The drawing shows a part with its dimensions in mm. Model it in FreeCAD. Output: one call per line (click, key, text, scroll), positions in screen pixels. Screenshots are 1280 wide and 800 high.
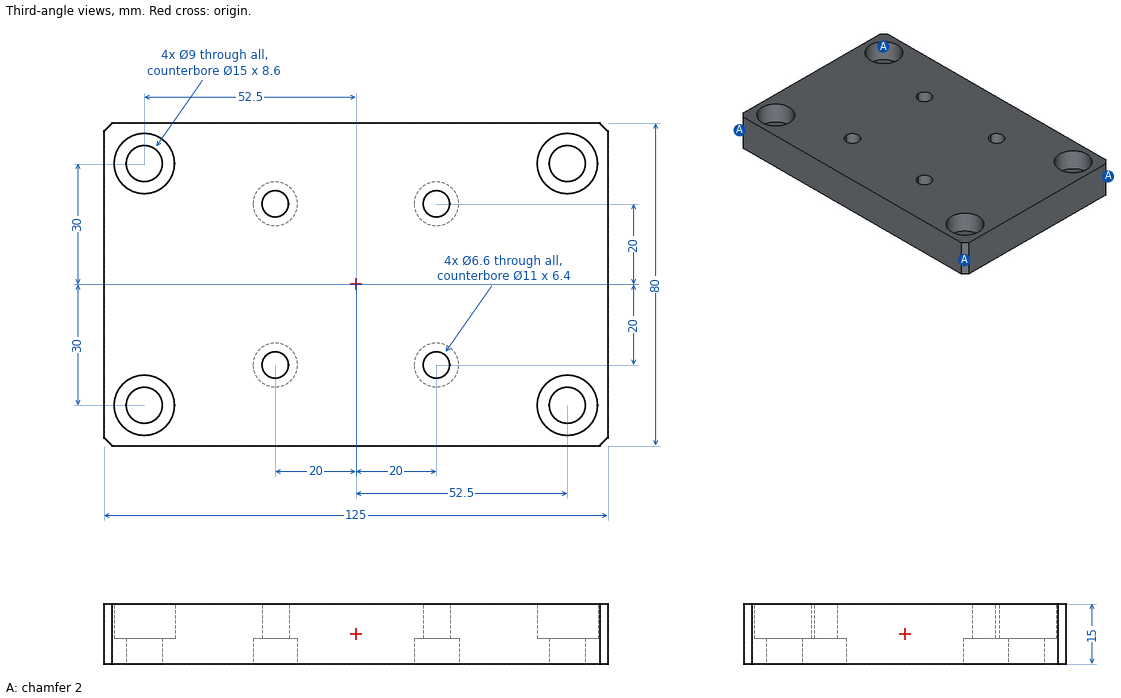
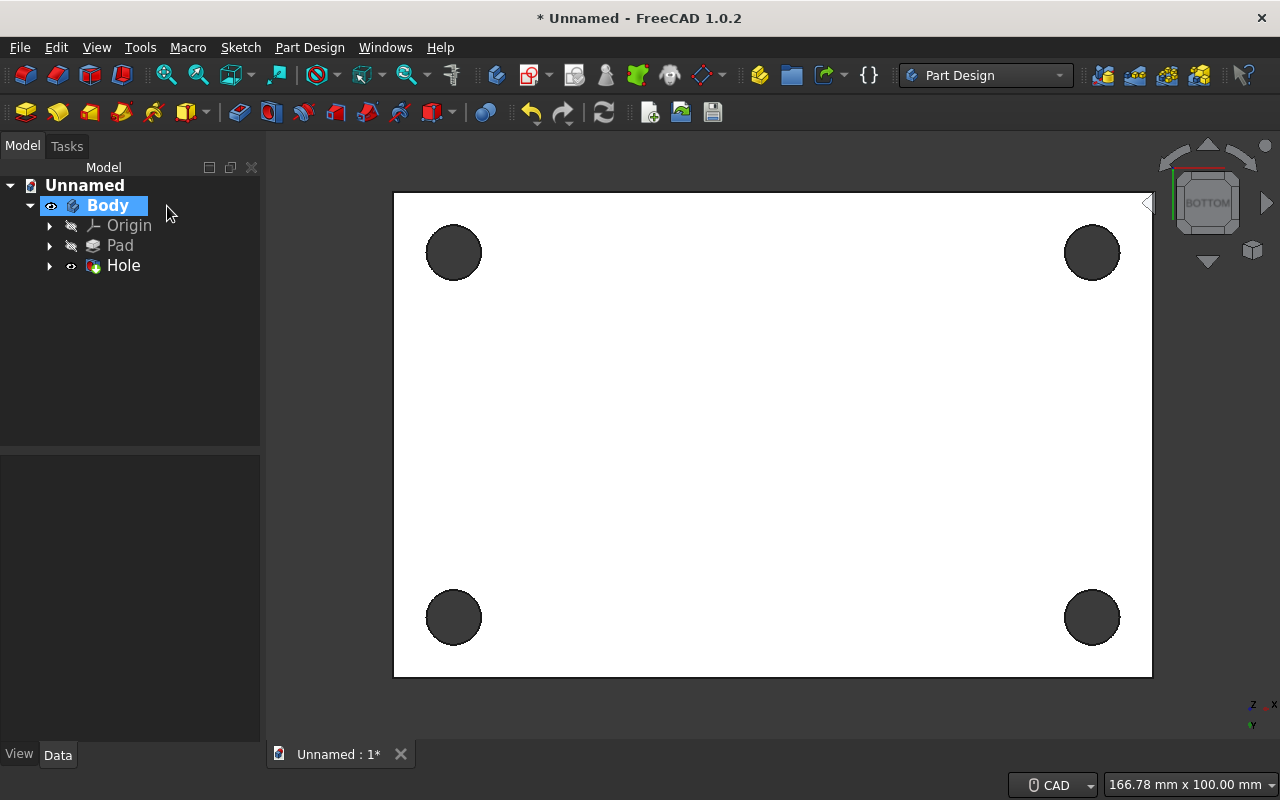
click(882, 434)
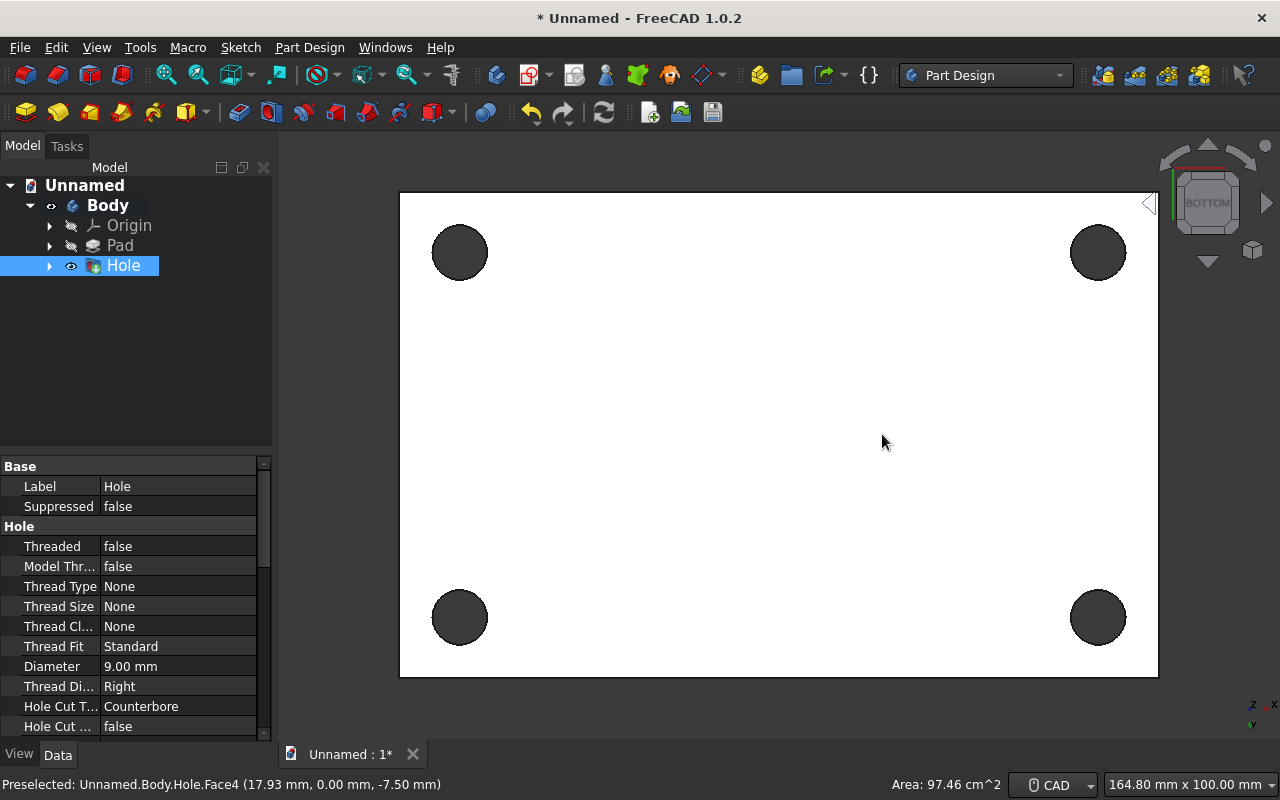
click(530, 76)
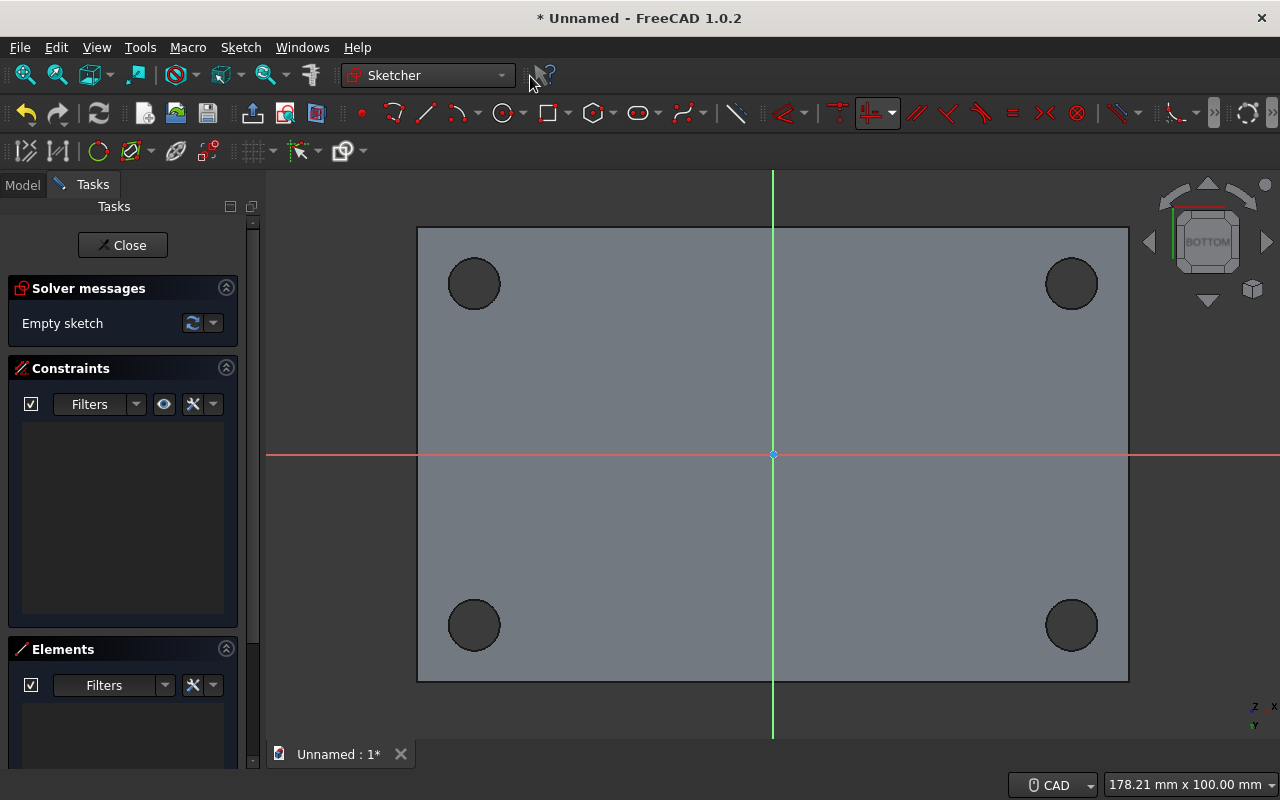
scroll(912, 455, up, 2)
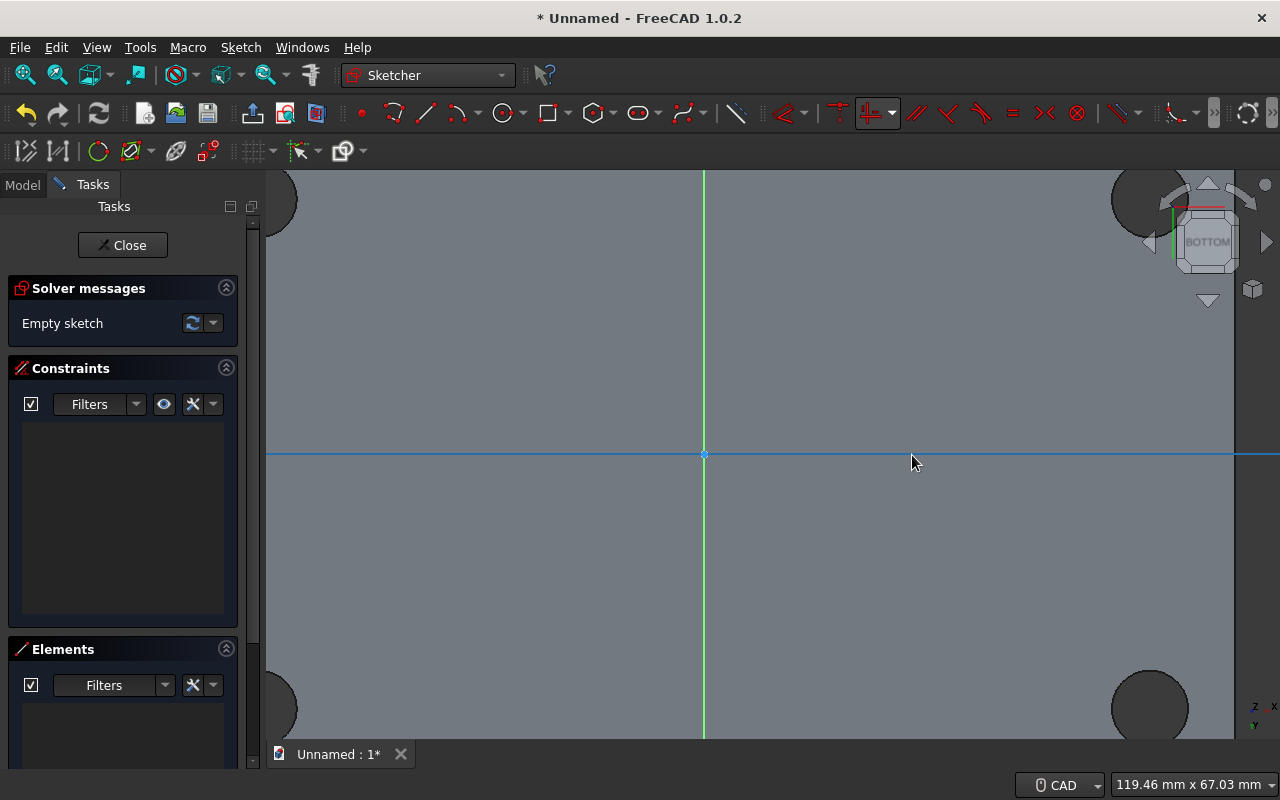
key(g)
key(c)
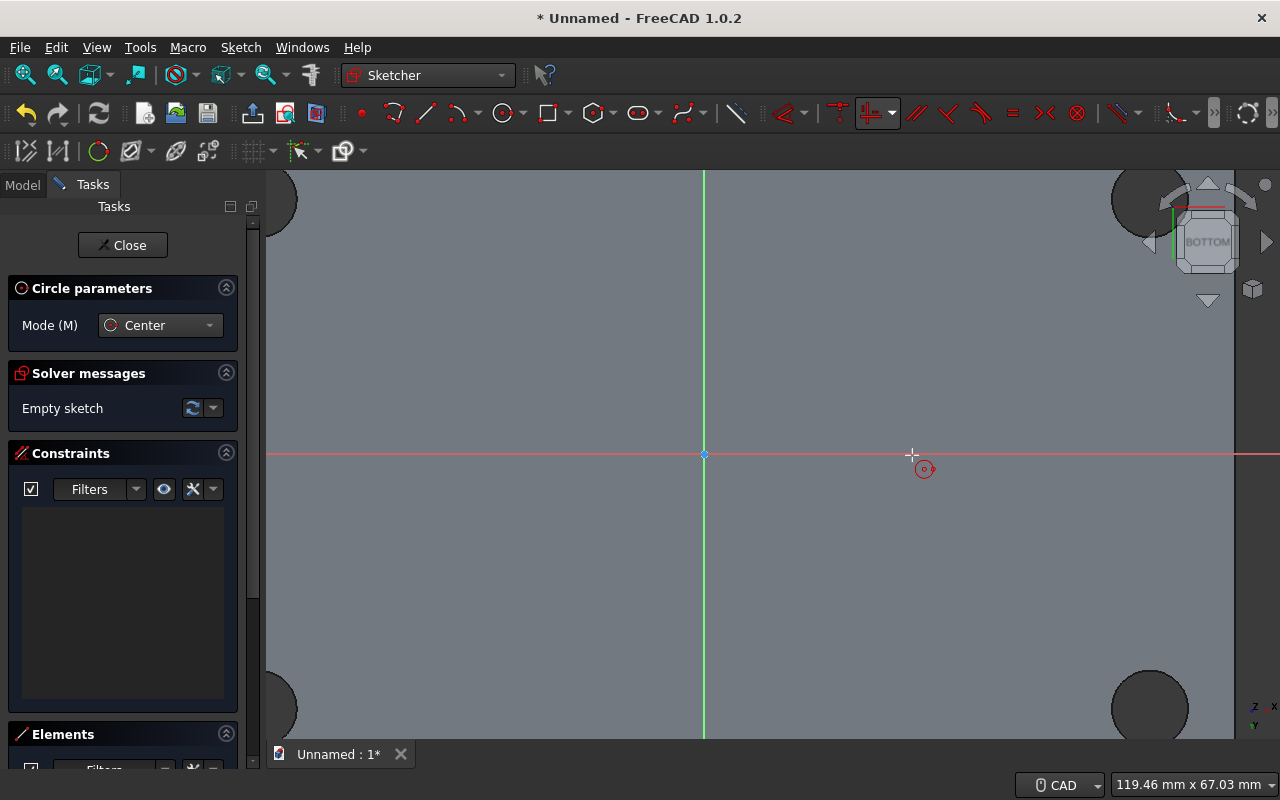
click(874, 284)
move(894, 264)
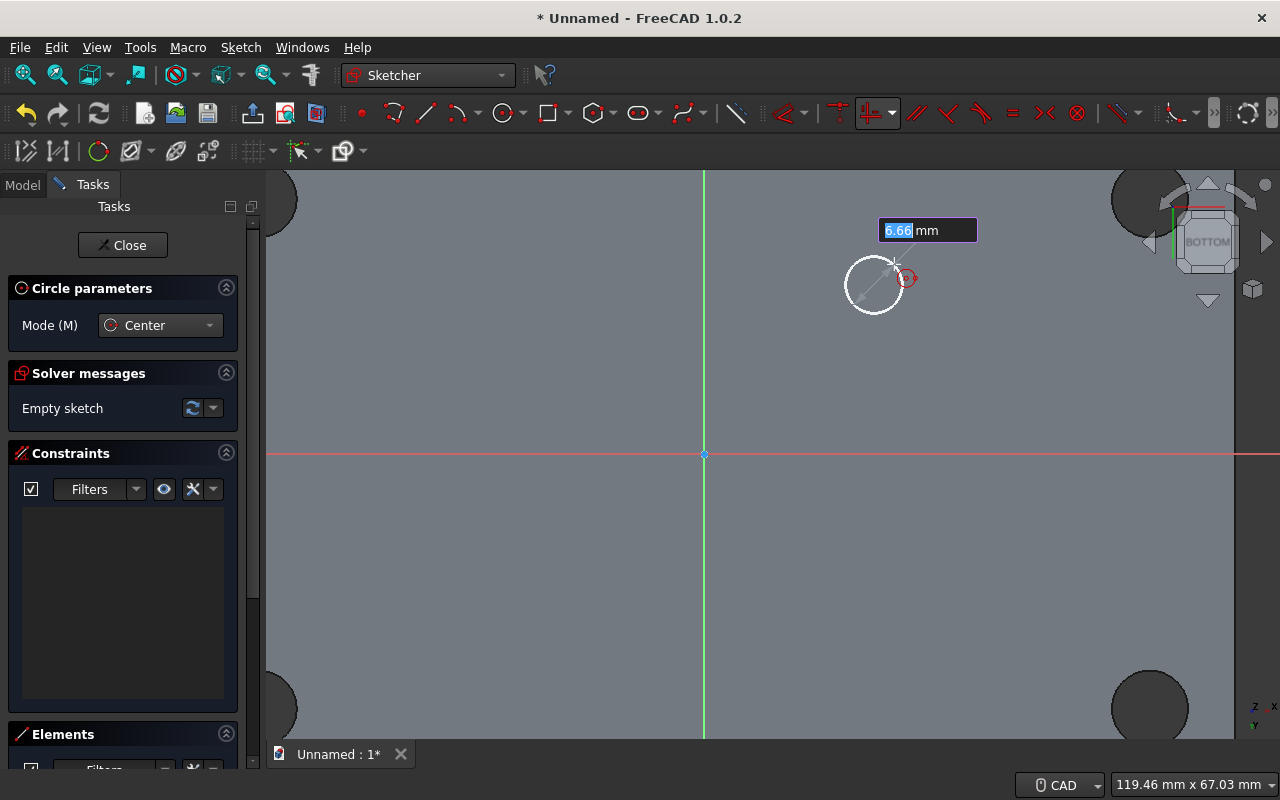
text(6.6)
key(Return)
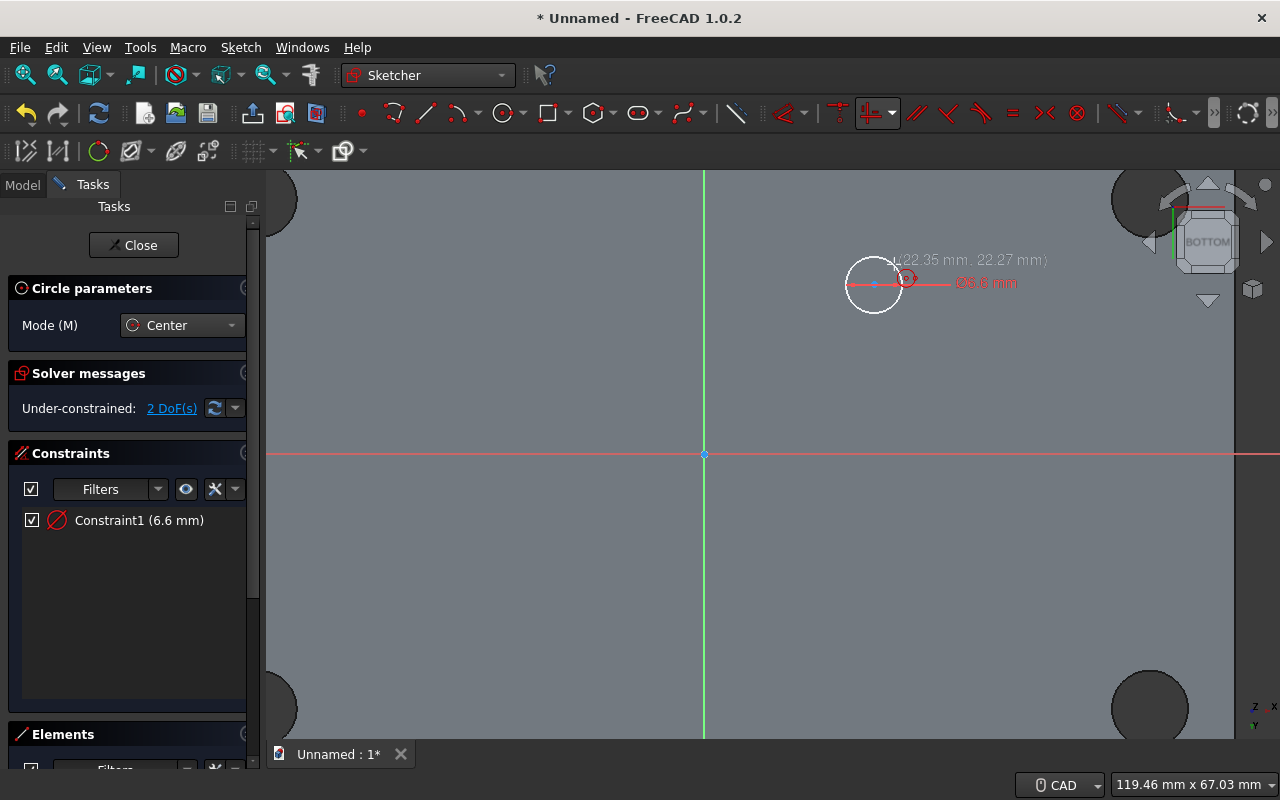
click(874, 624)
move(894, 604)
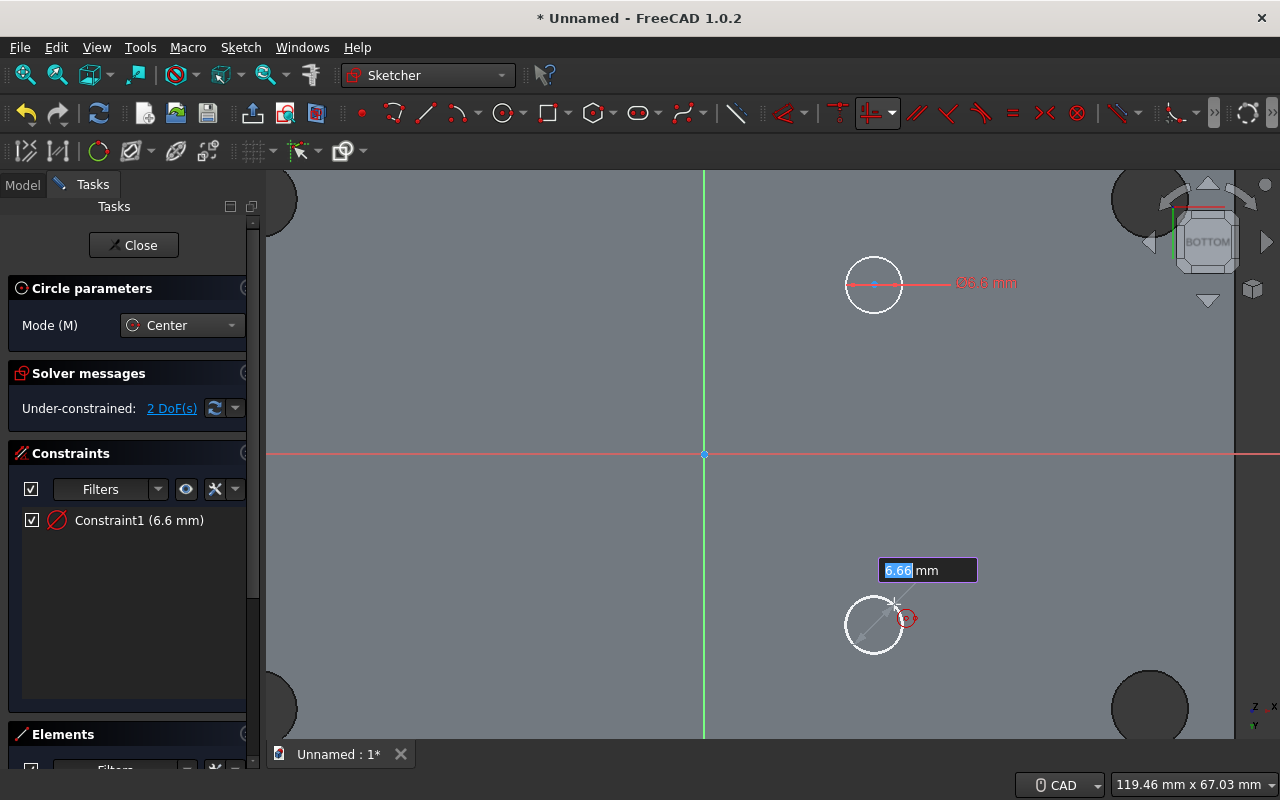
text(6.6)
key(Return)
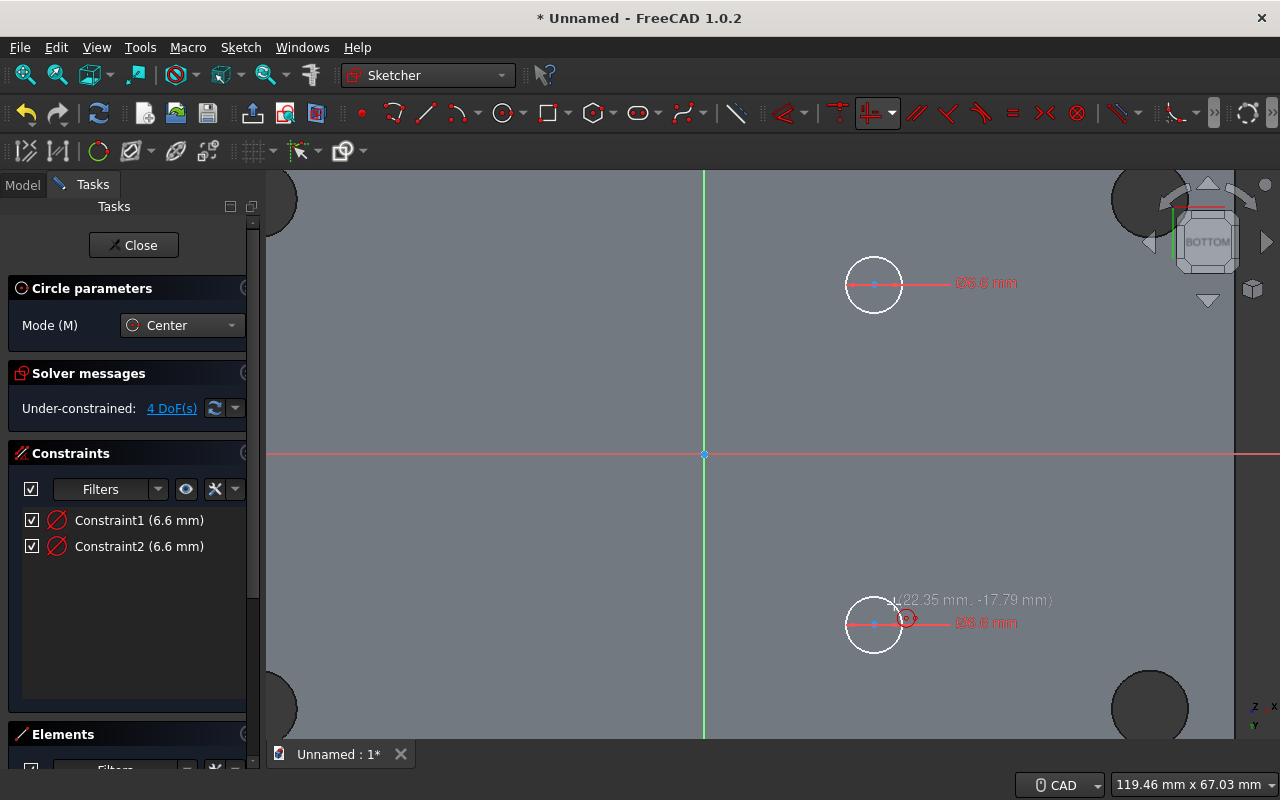
click(535, 284)
move(554, 264)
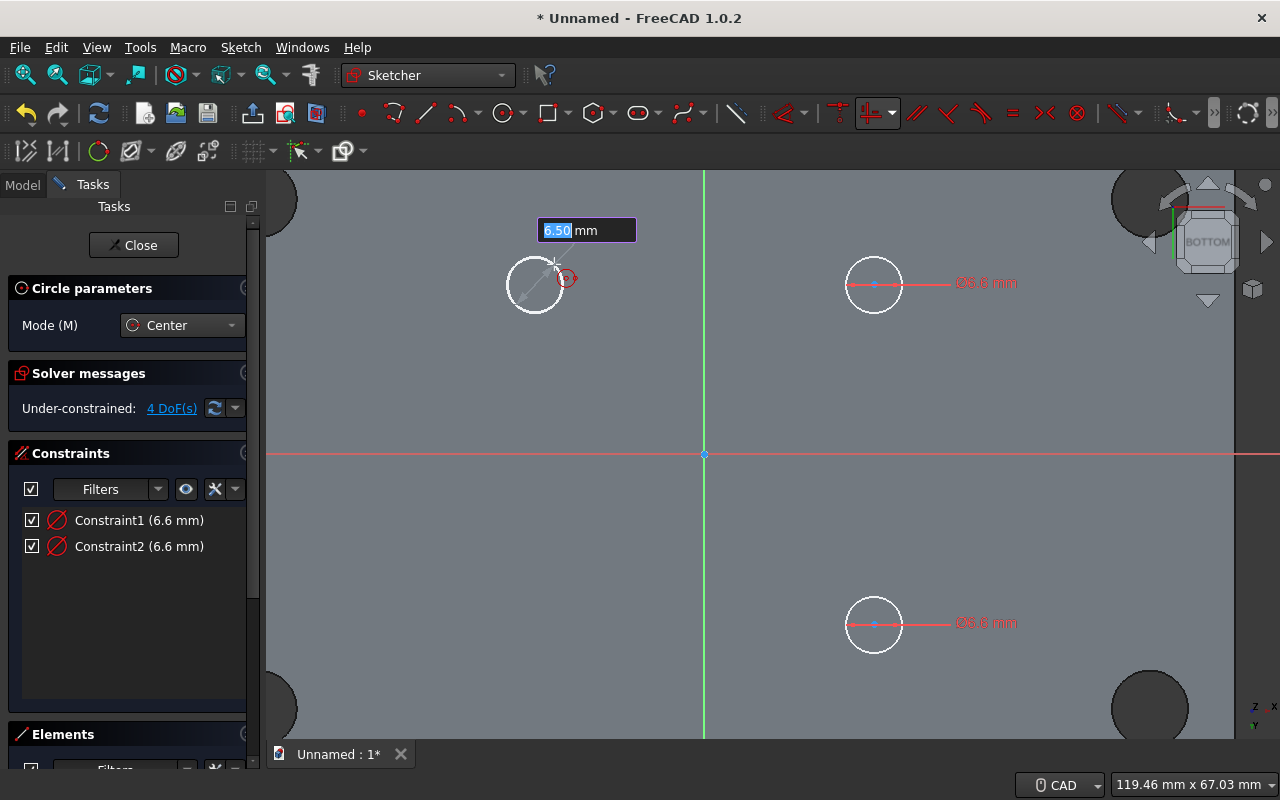
text(6.6)
key(Return)